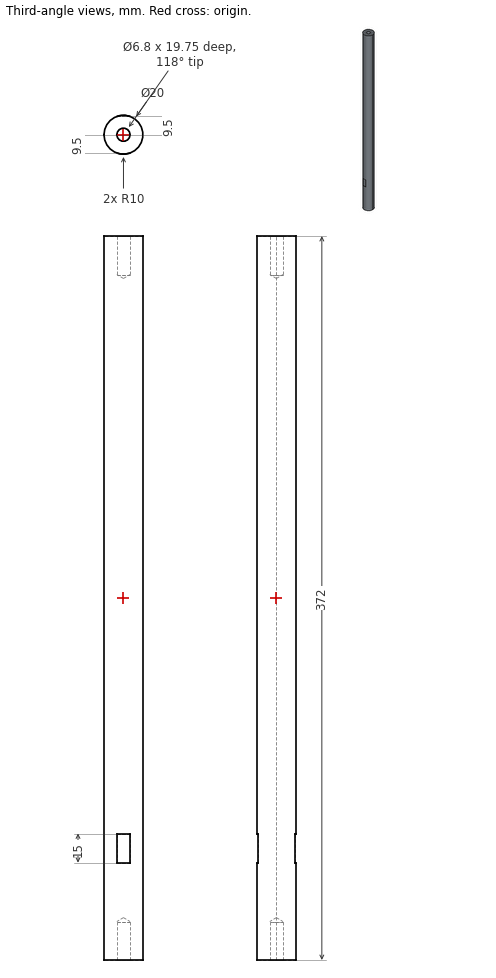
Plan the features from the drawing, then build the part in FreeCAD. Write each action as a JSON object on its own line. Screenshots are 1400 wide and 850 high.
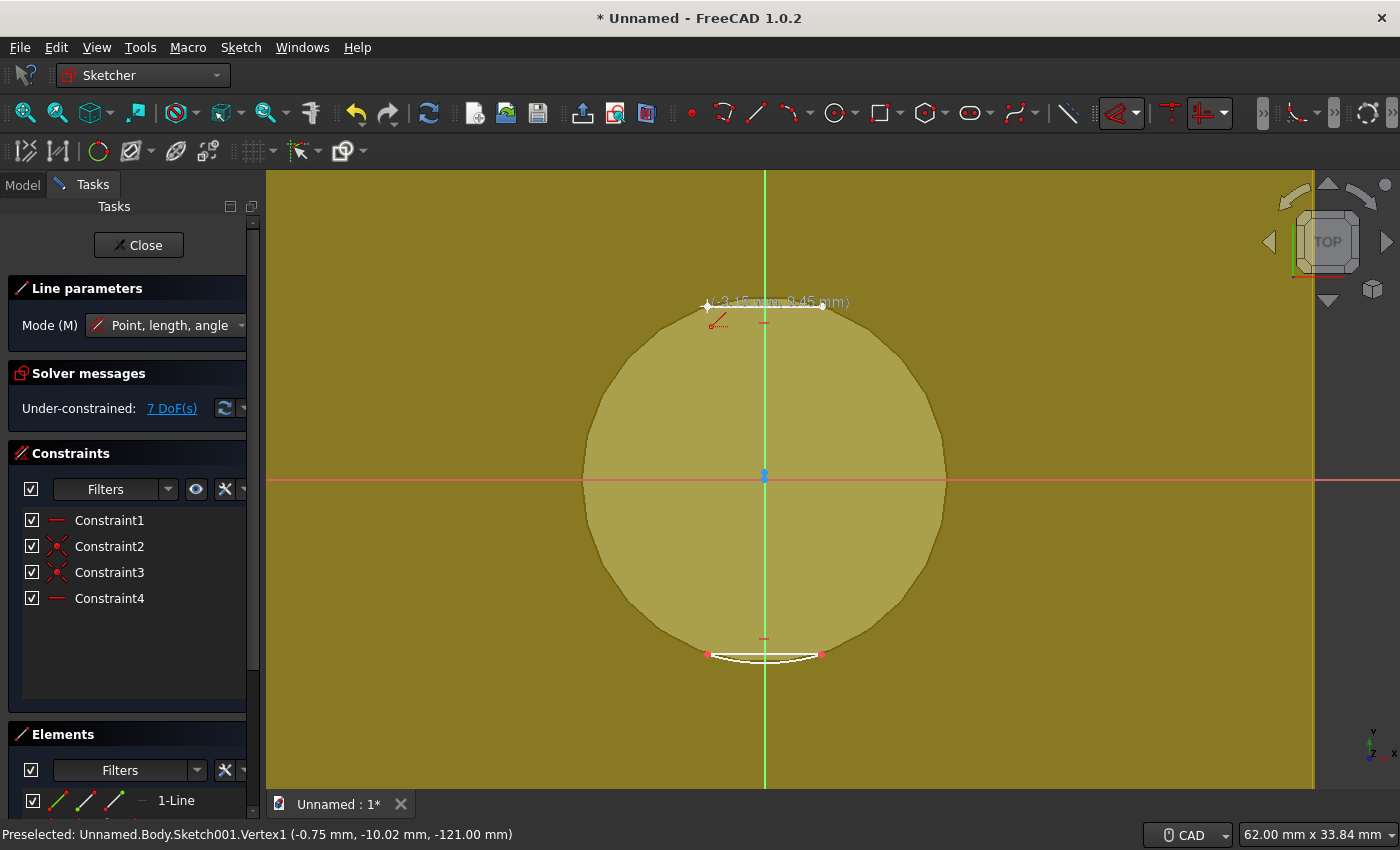
{"action": "left_click", "coordinate": [790, 114]}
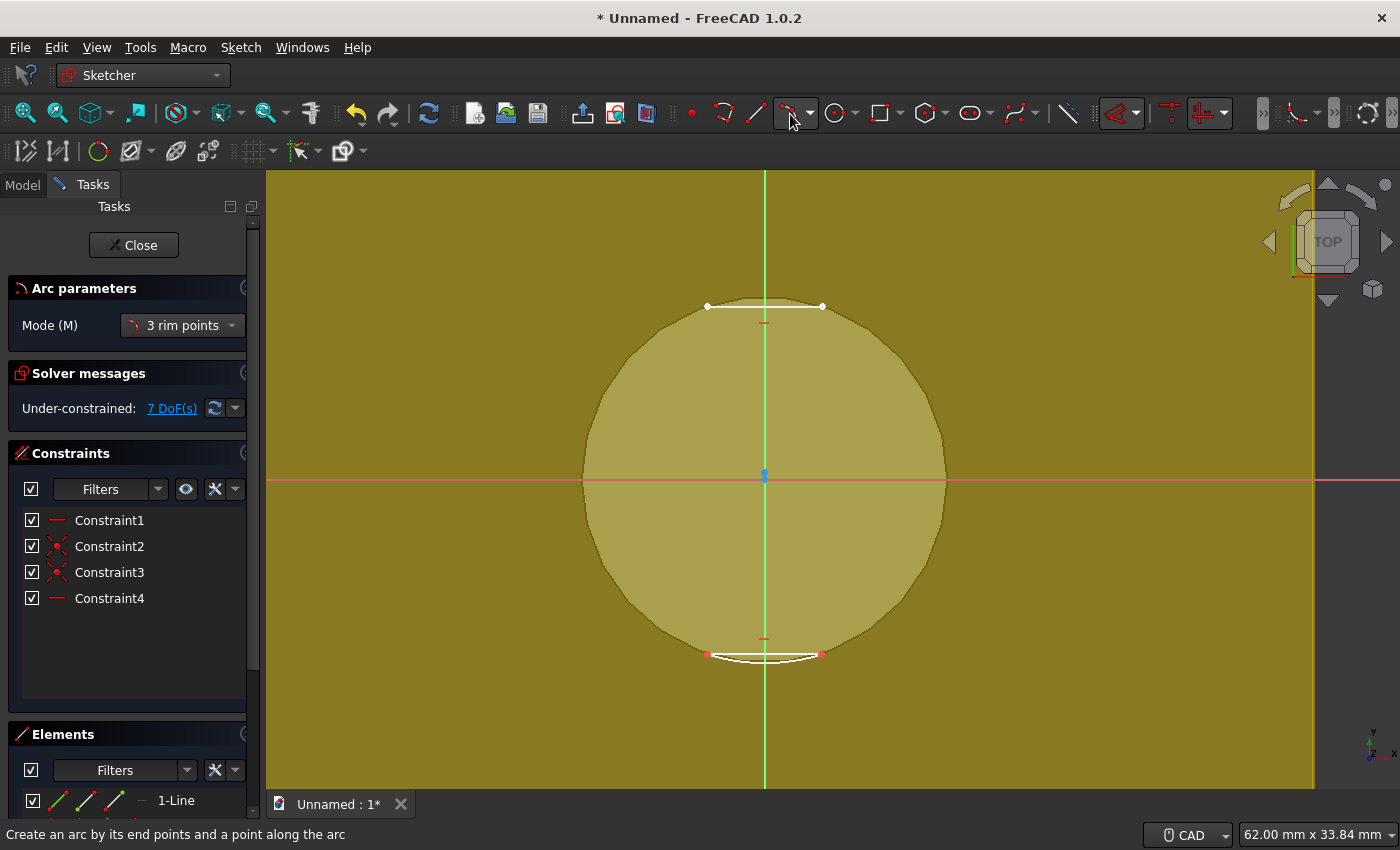
{"action": "left_click", "coordinate": [707, 307]}
{"action": "left_click", "coordinate": [822, 307]}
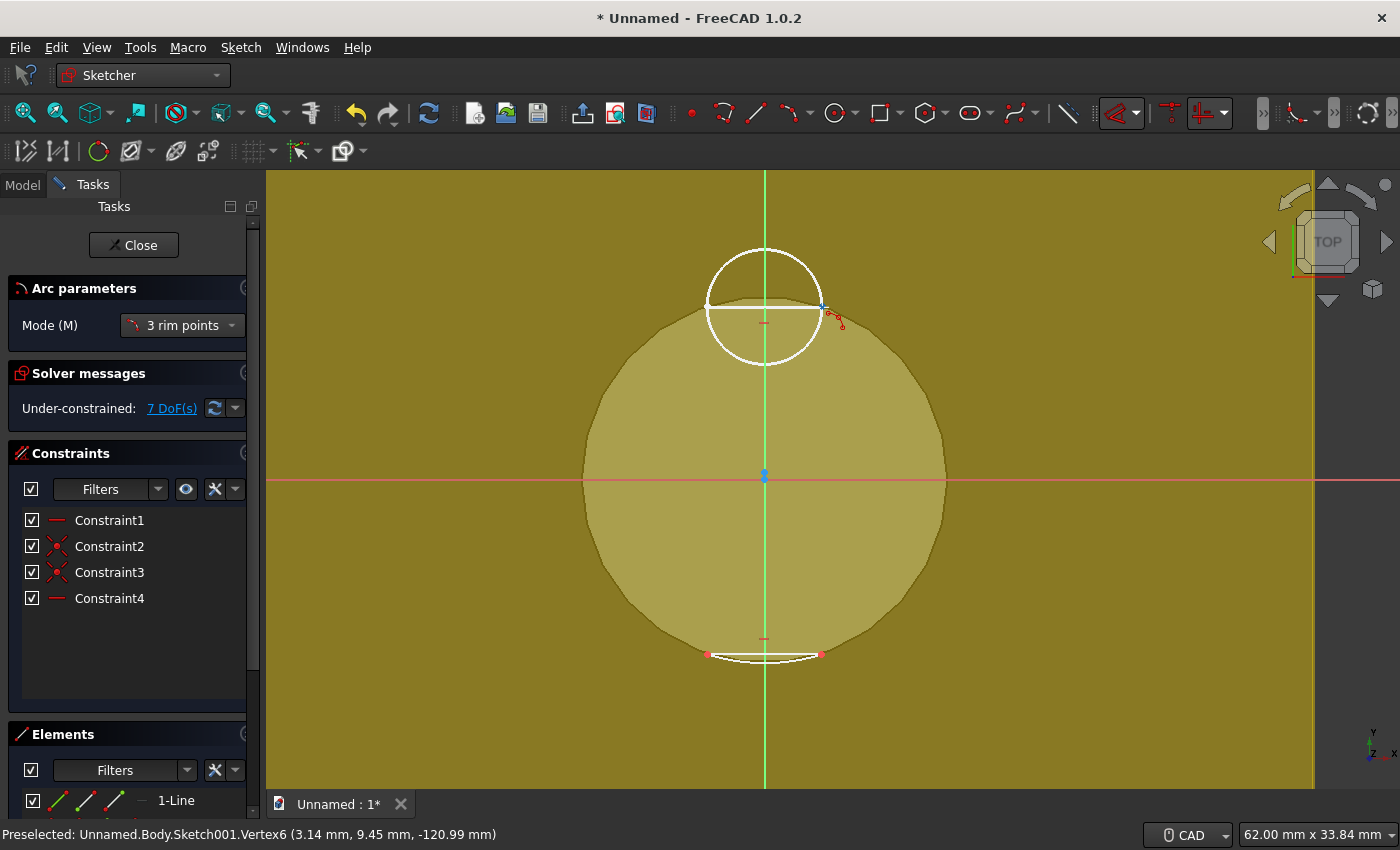
{"action": "scroll", "coordinate": [776, 297], "scroll_direction": "up", "scroll_amount": 3}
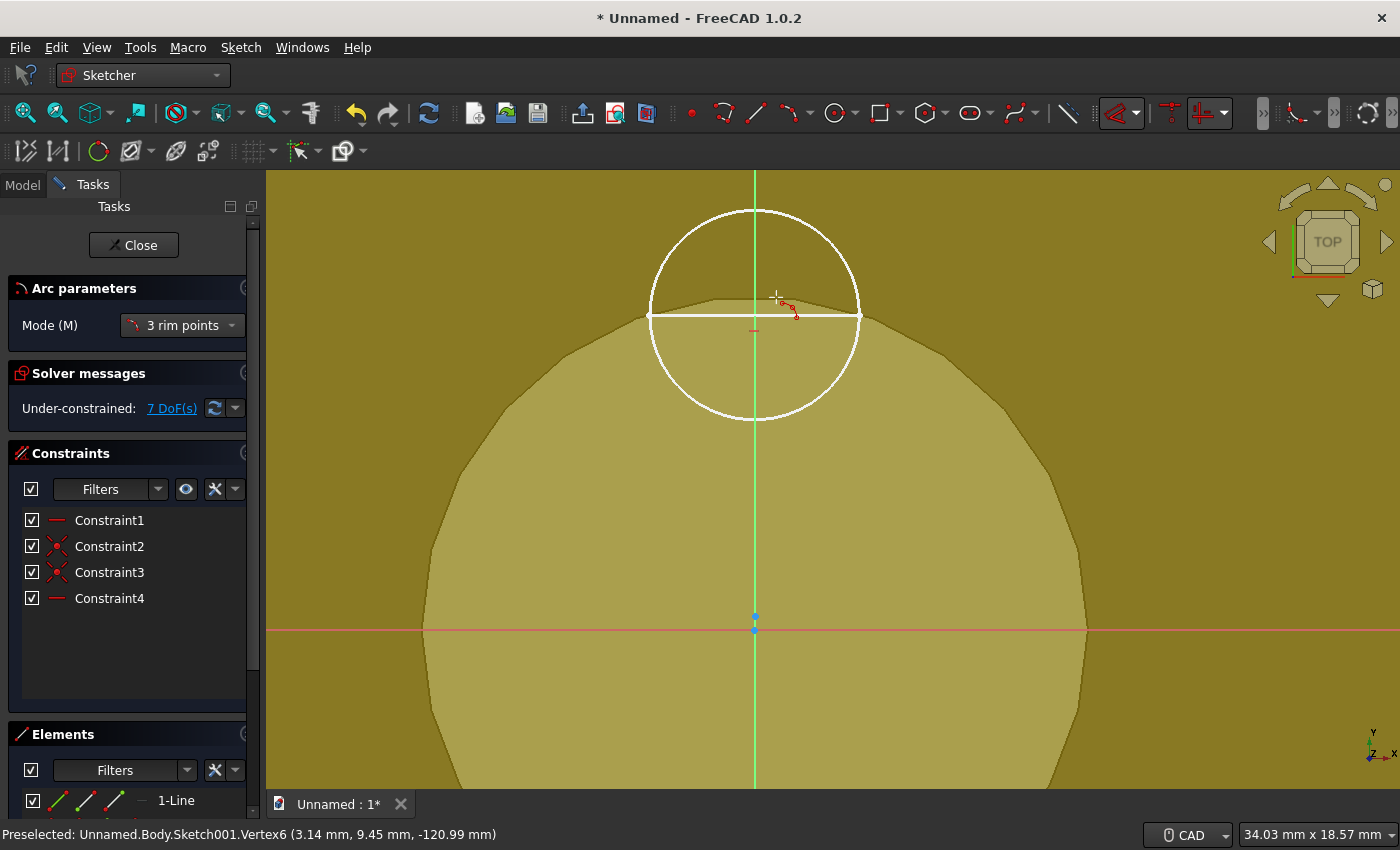
{"action": "left_click", "coordinate": [776, 297]}
{"action": "key", "text": "Escape"}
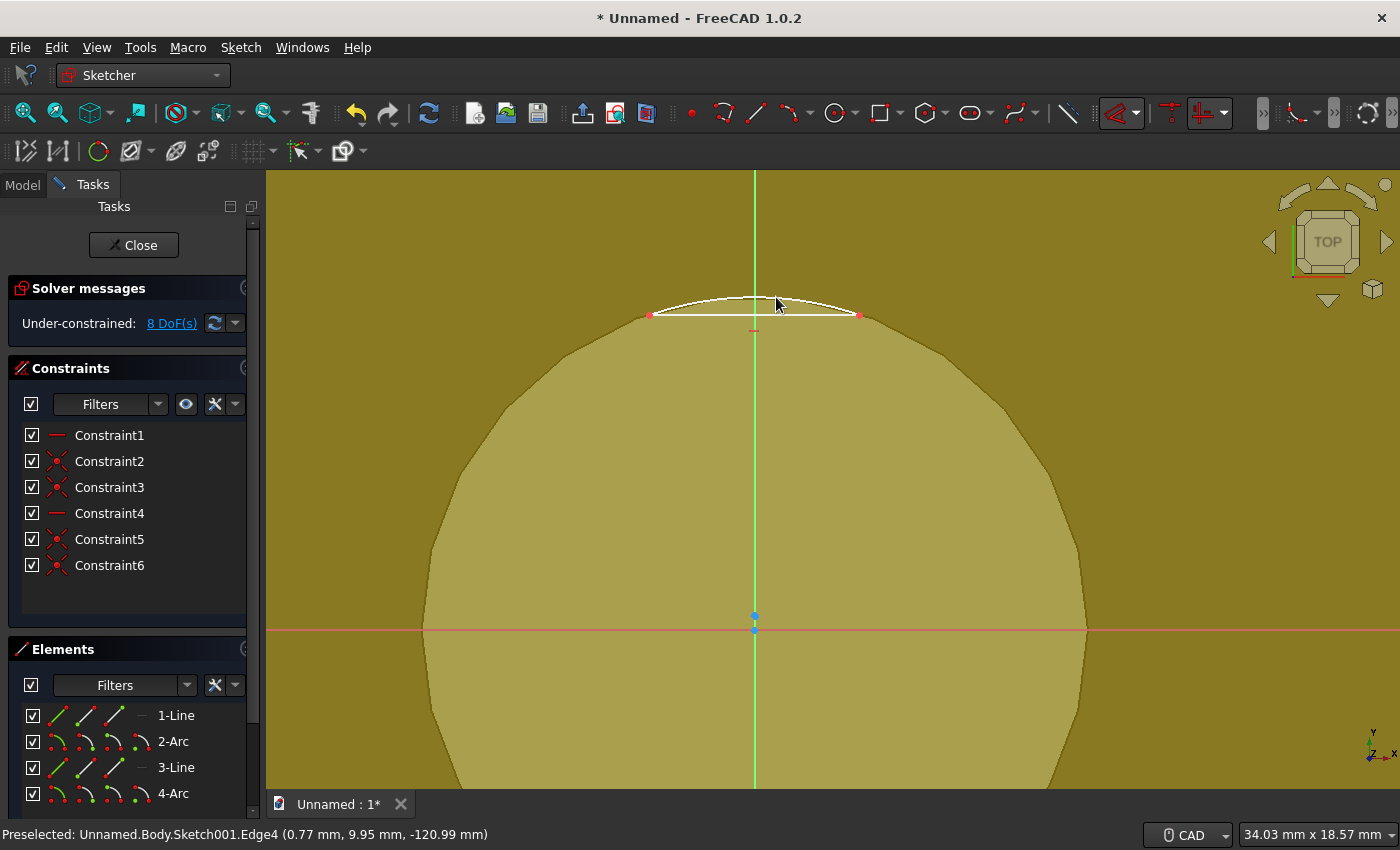
{"action": "scroll", "coordinate": [776, 296], "scroll_direction": "down", "scroll_amount": 3}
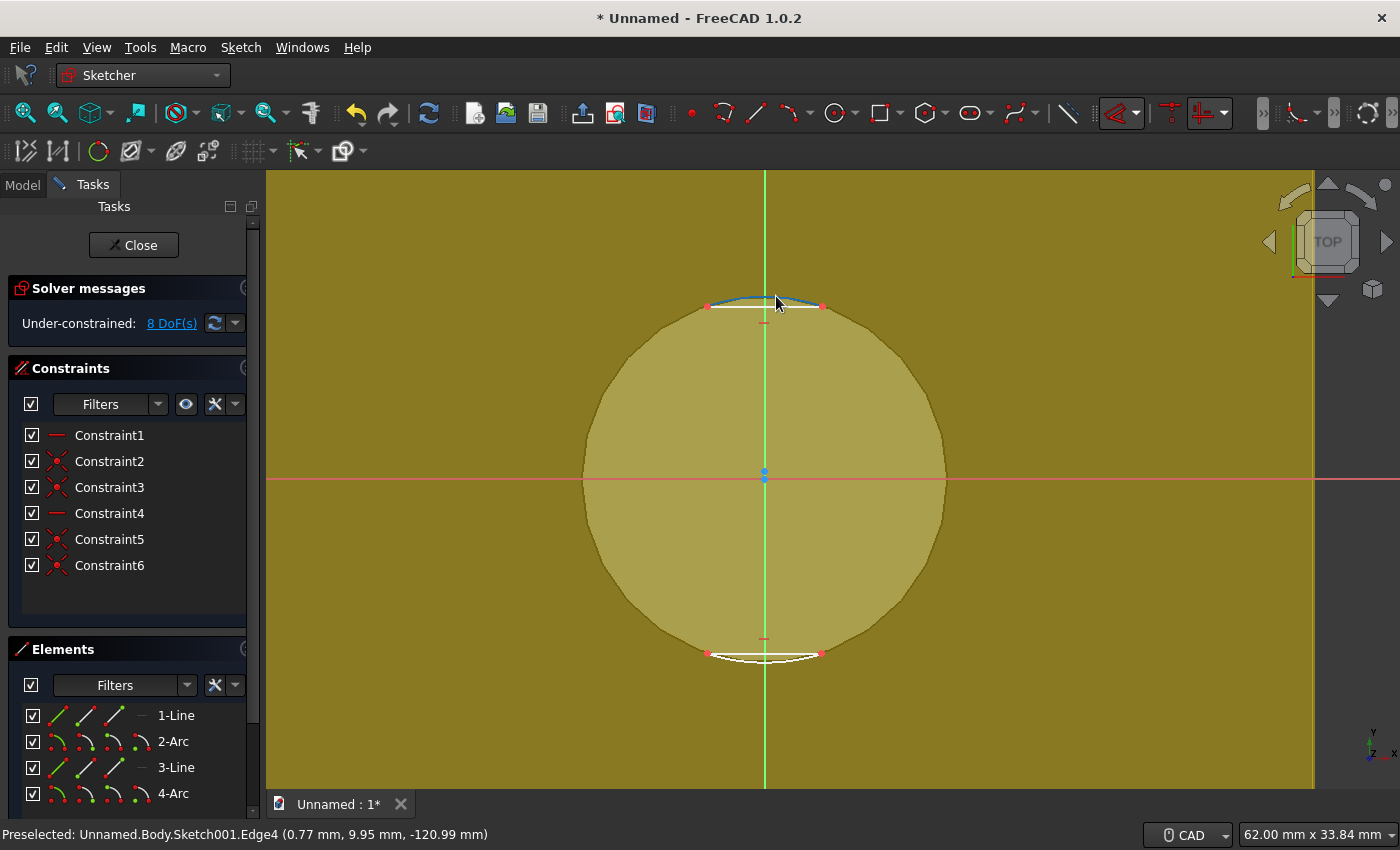
{"action": "scroll", "coordinate": [742, 661], "scroll_direction": "up", "scroll_amount": 4}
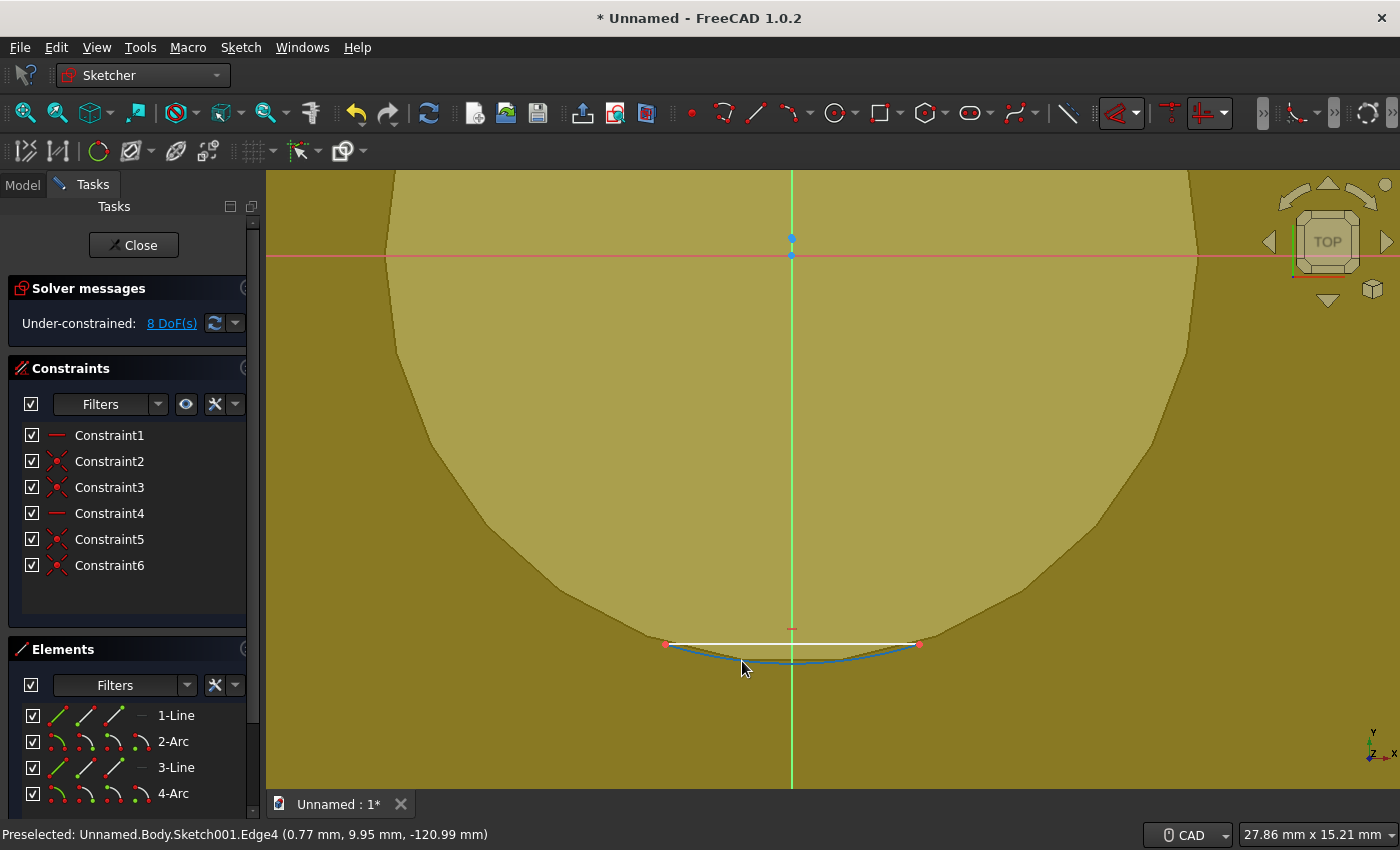
{"action": "left_click", "coordinate": [741, 661]}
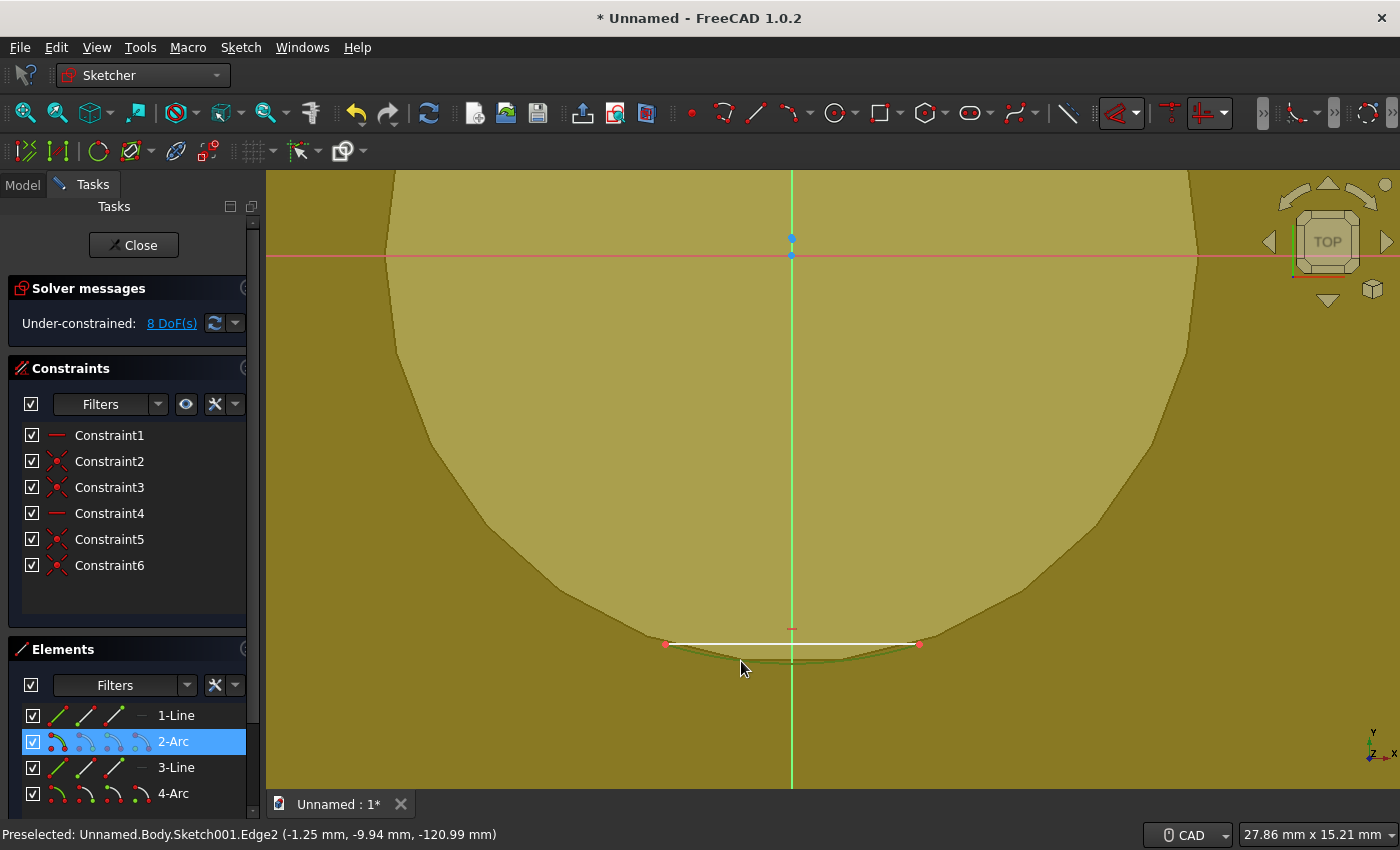
{"action": "scroll", "coordinate": [742, 662], "scroll_direction": "down", "scroll_amount": 4}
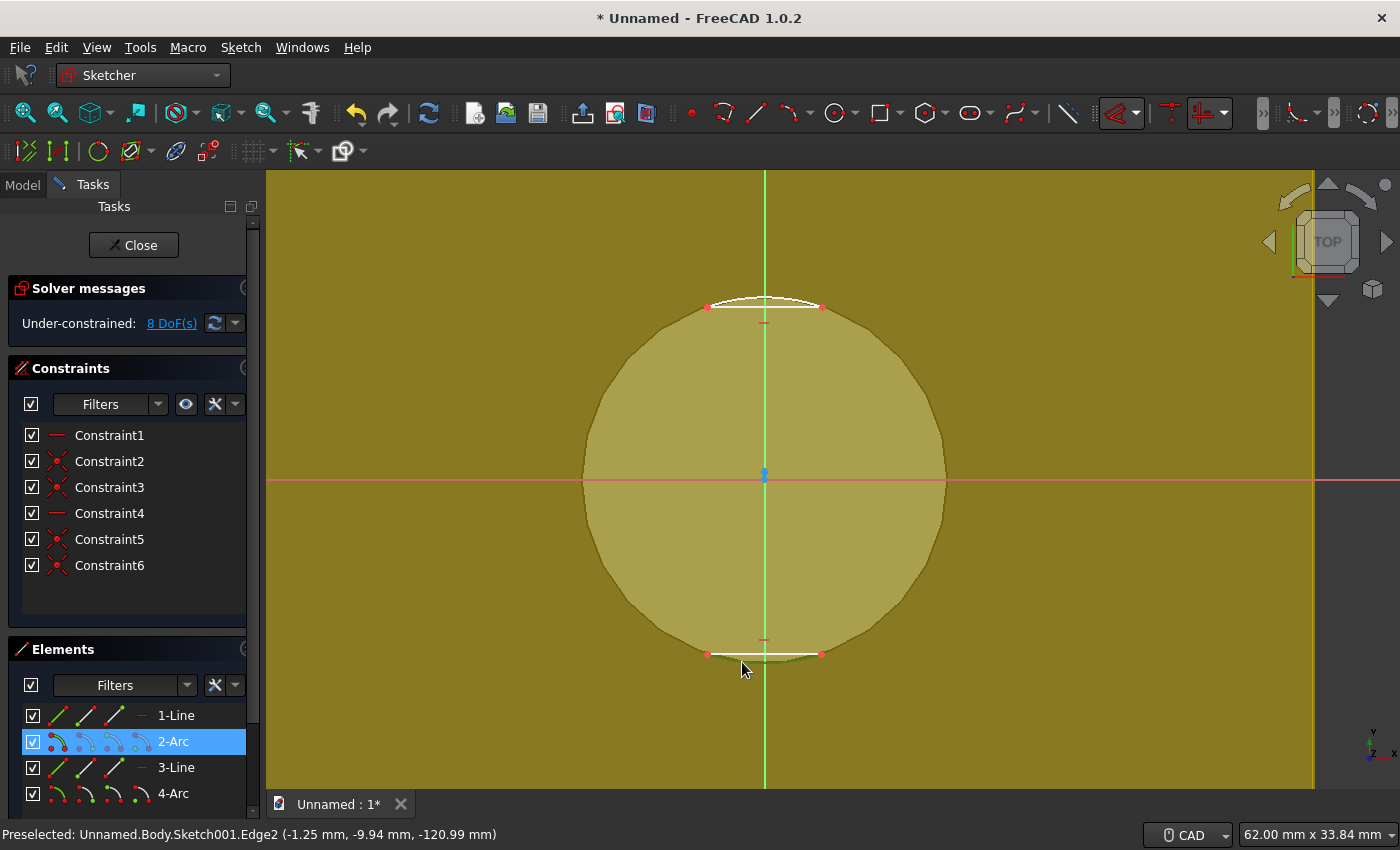
{"action": "scroll", "coordinate": [788, 299], "scroll_direction": "up", "scroll_amount": 3}